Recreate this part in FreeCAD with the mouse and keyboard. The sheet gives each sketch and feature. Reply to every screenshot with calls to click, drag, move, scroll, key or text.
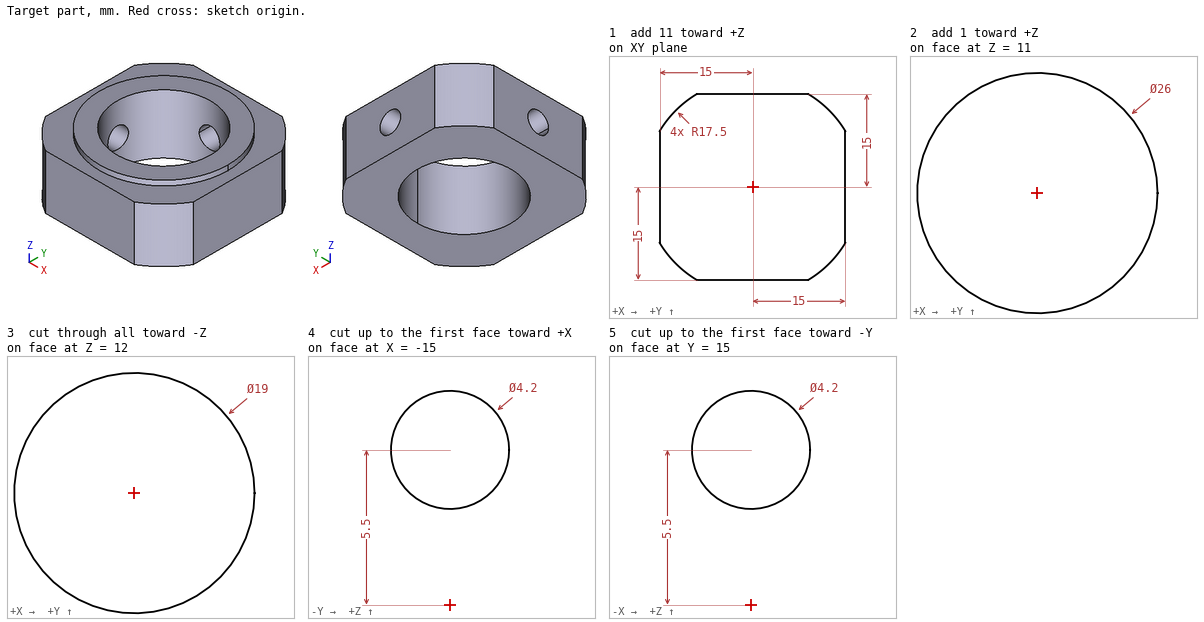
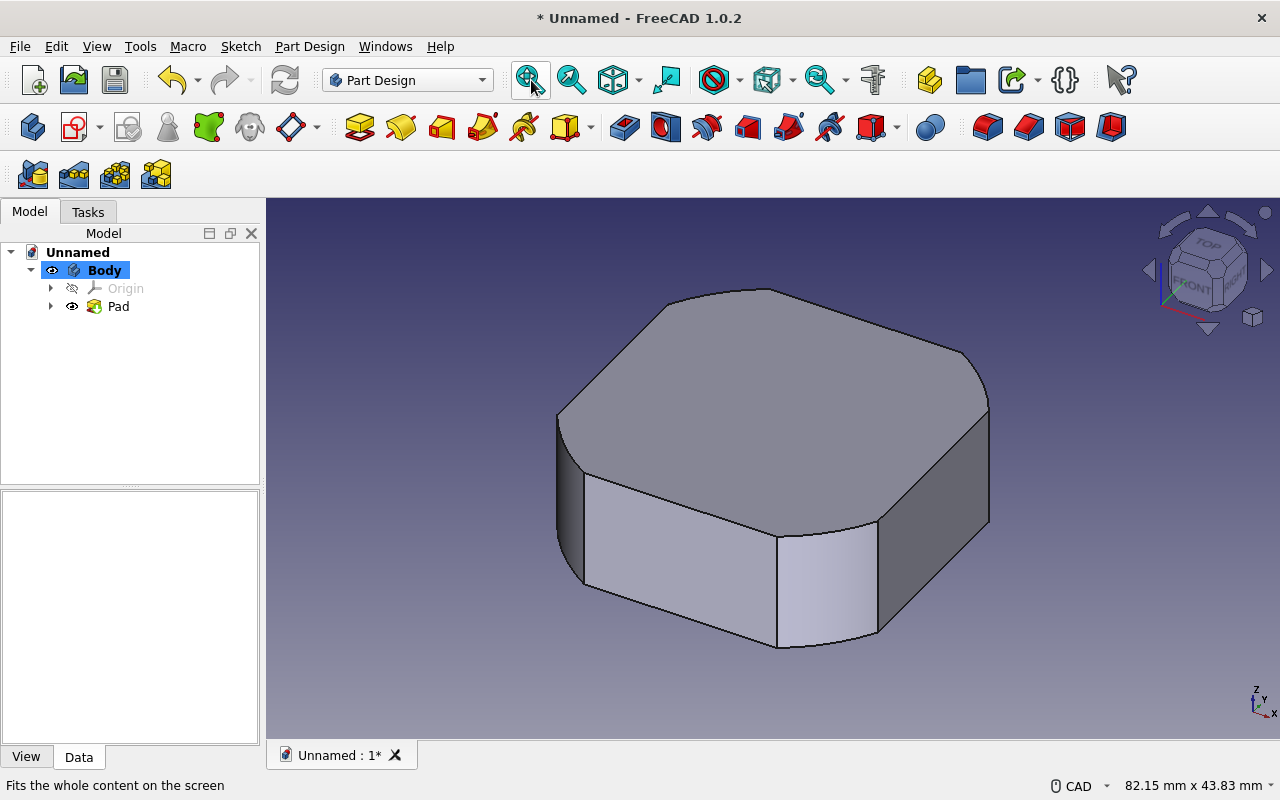
click(773, 412)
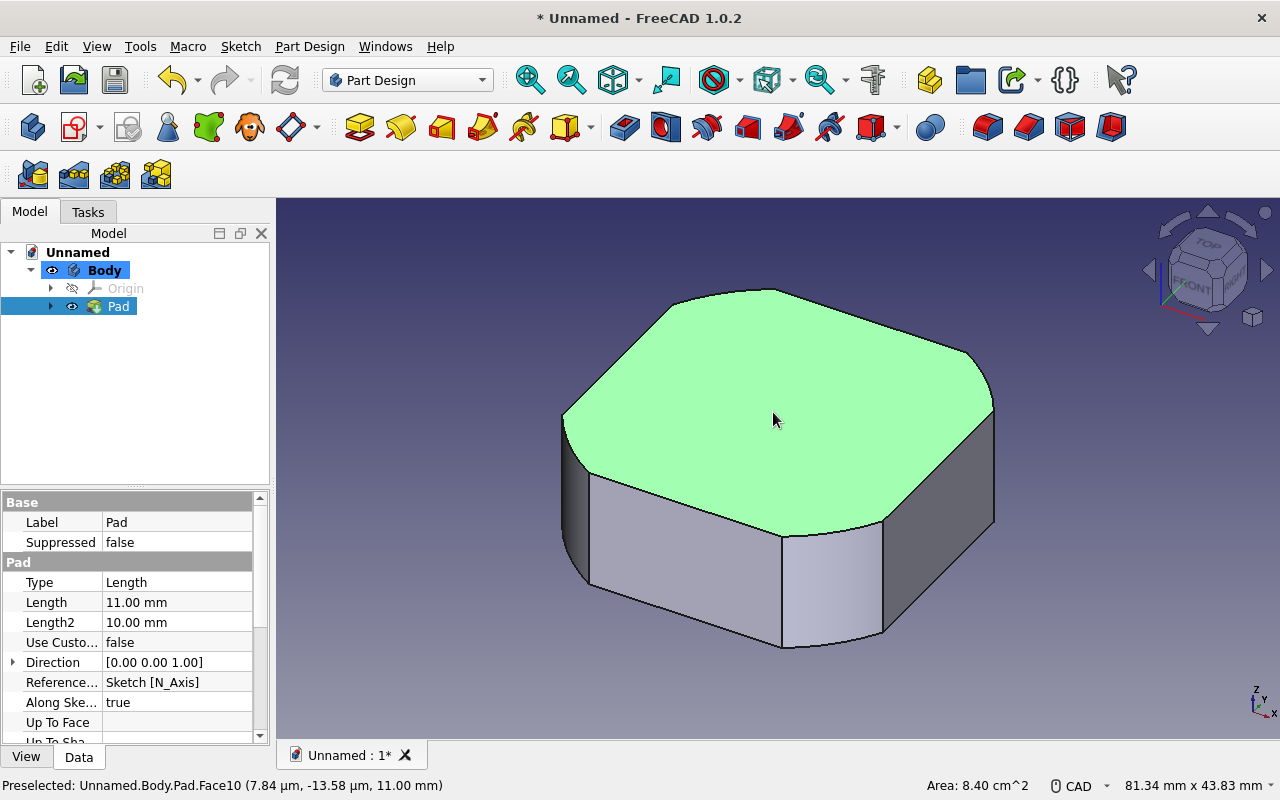
click(74, 128)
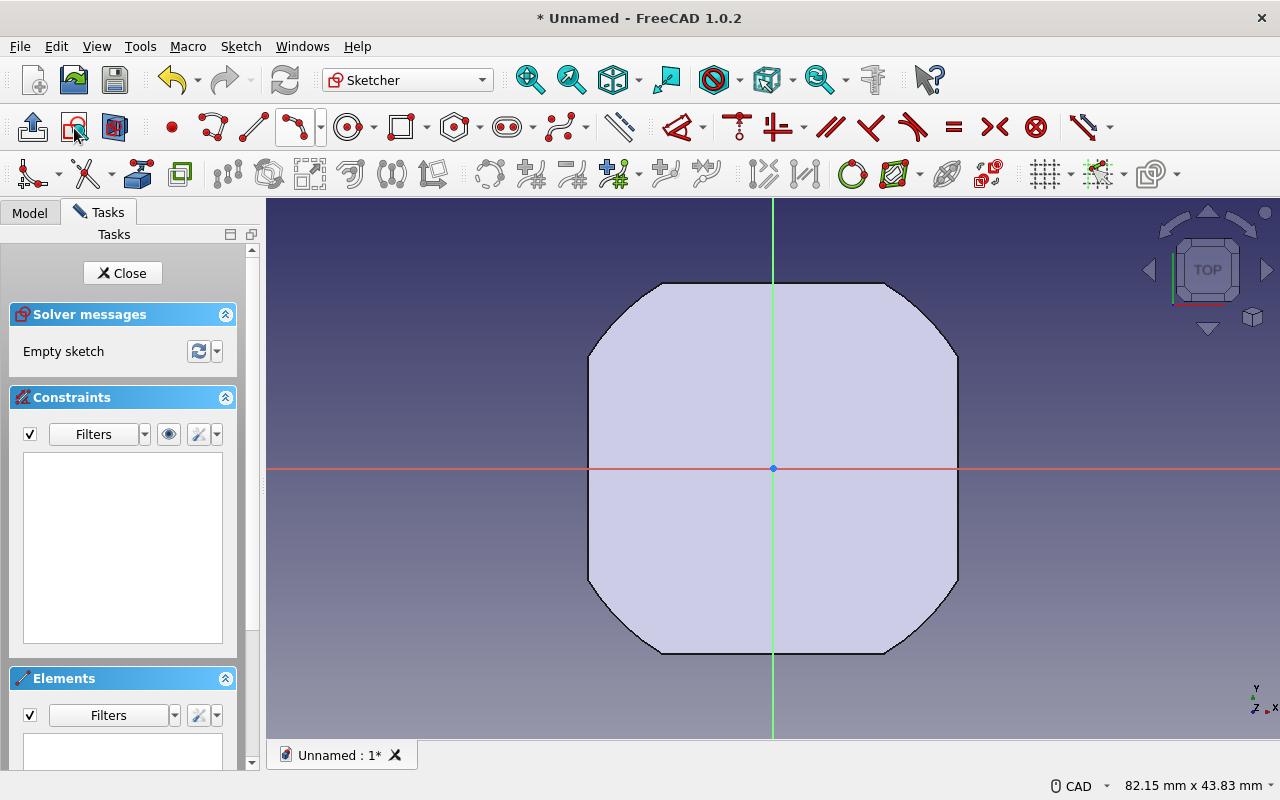
click(348, 128)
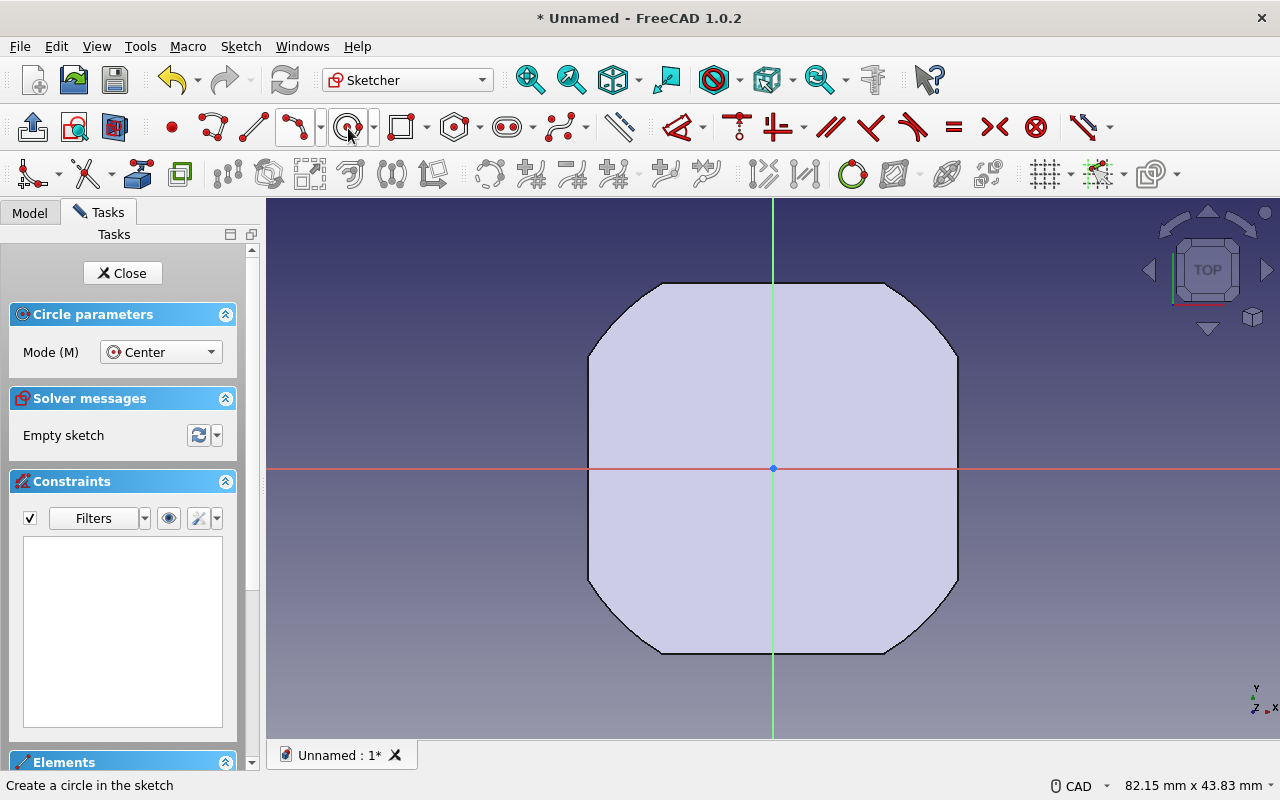
click(773, 468)
click(886, 355)
key(Escape)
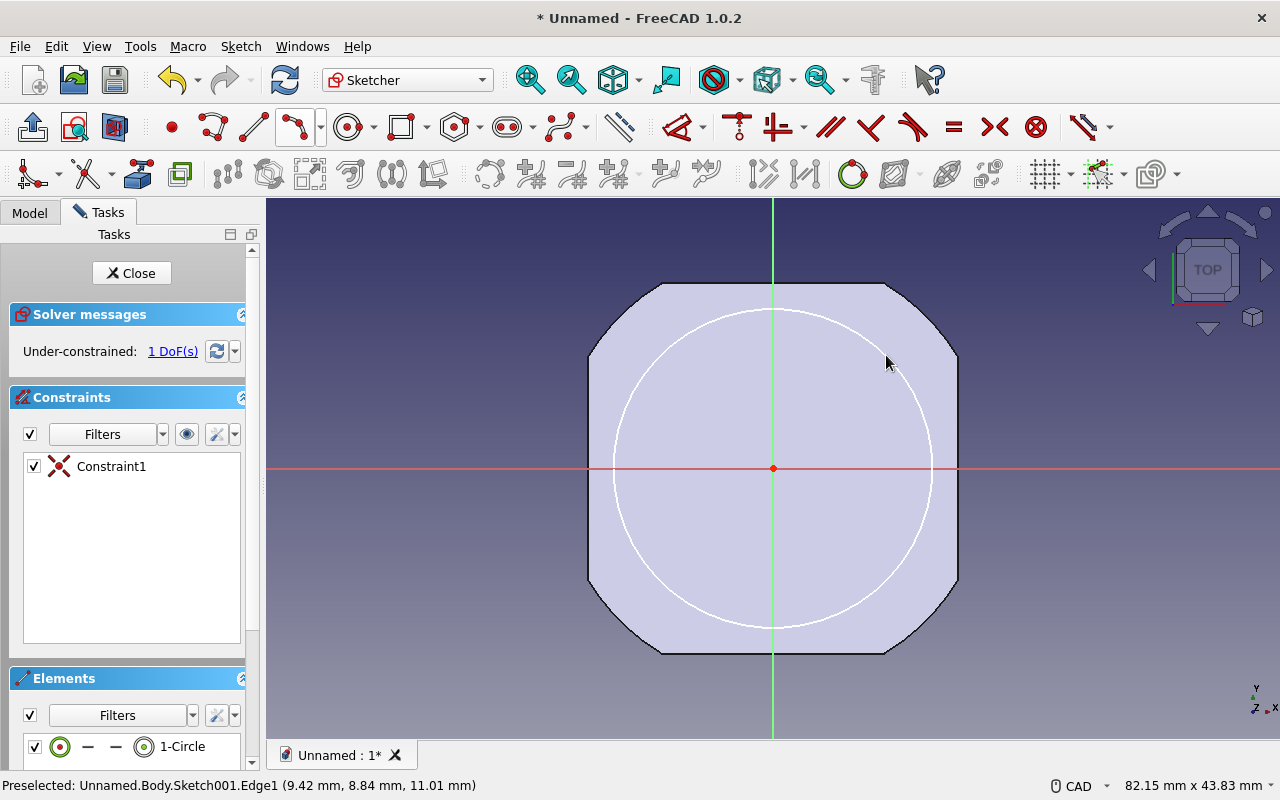
click(676, 128)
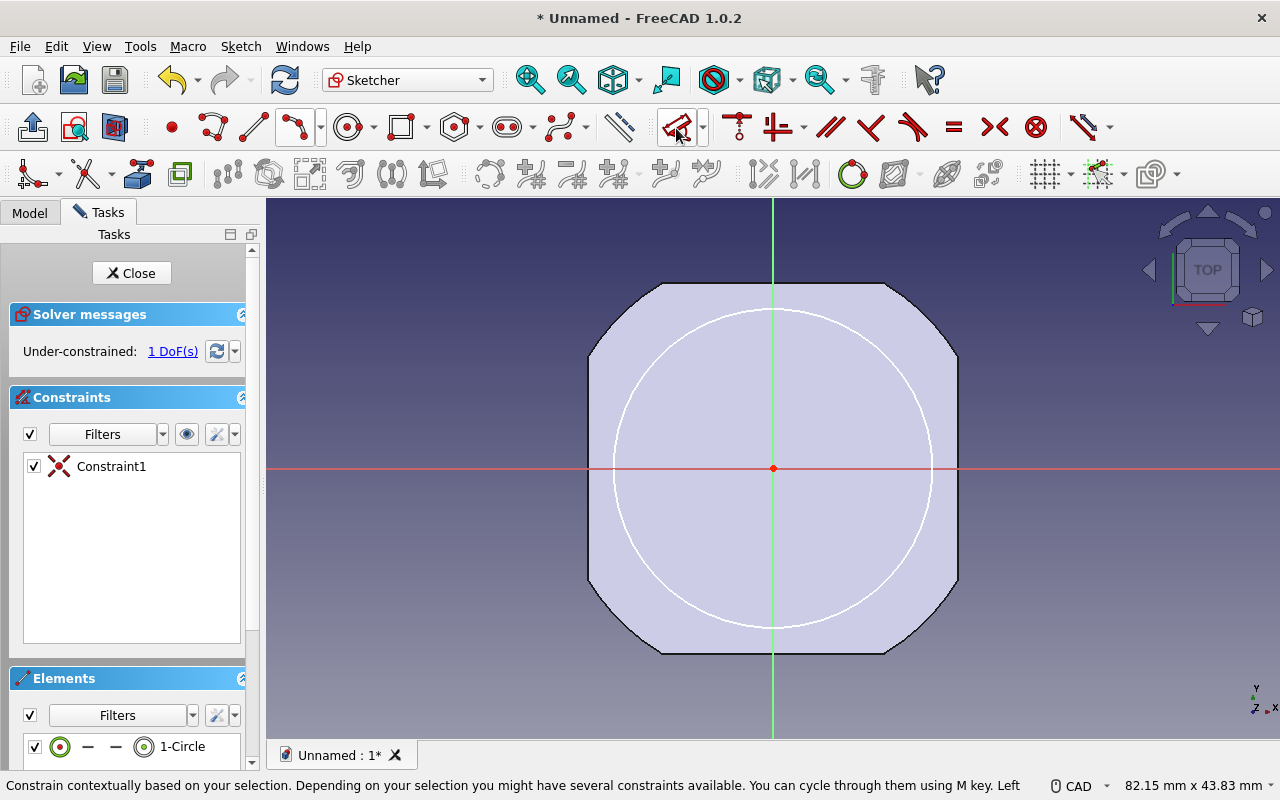
click(885, 355)
click(907, 332)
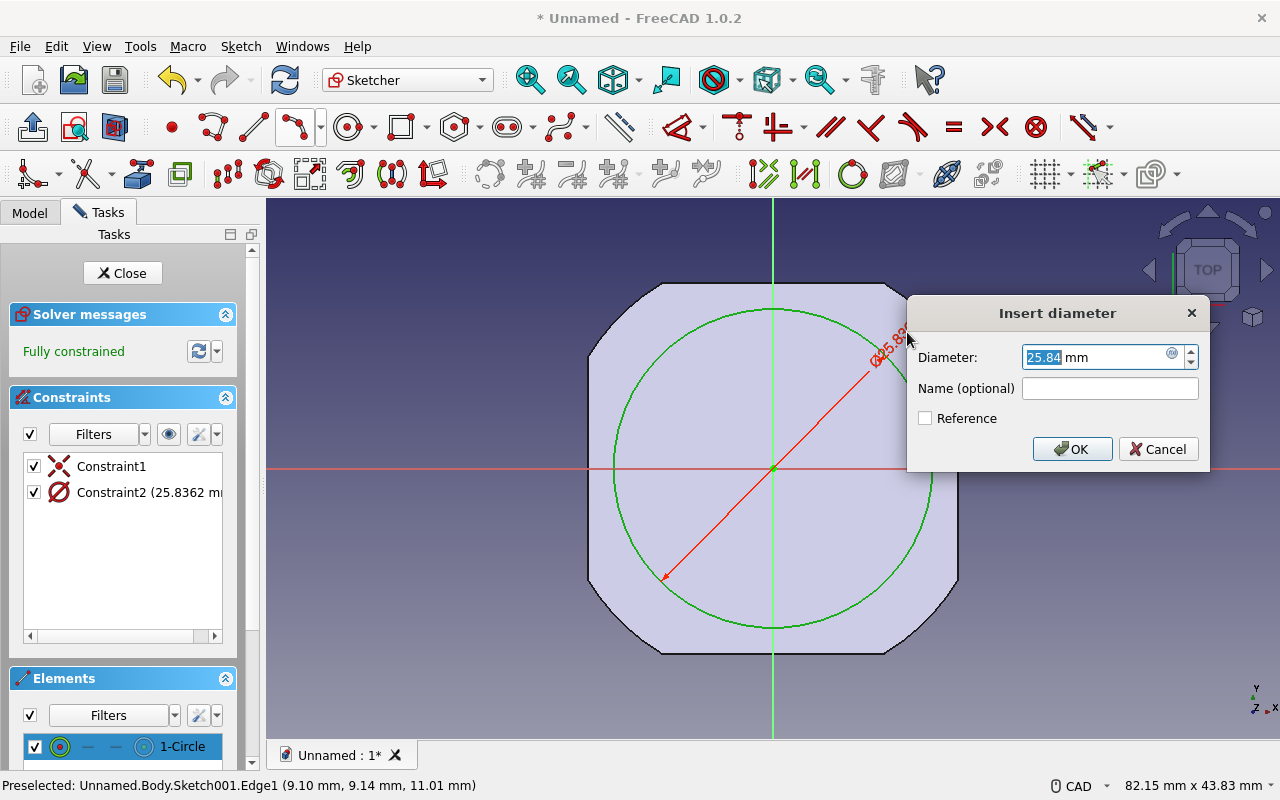
text(26)
key(Return)
key(Escape)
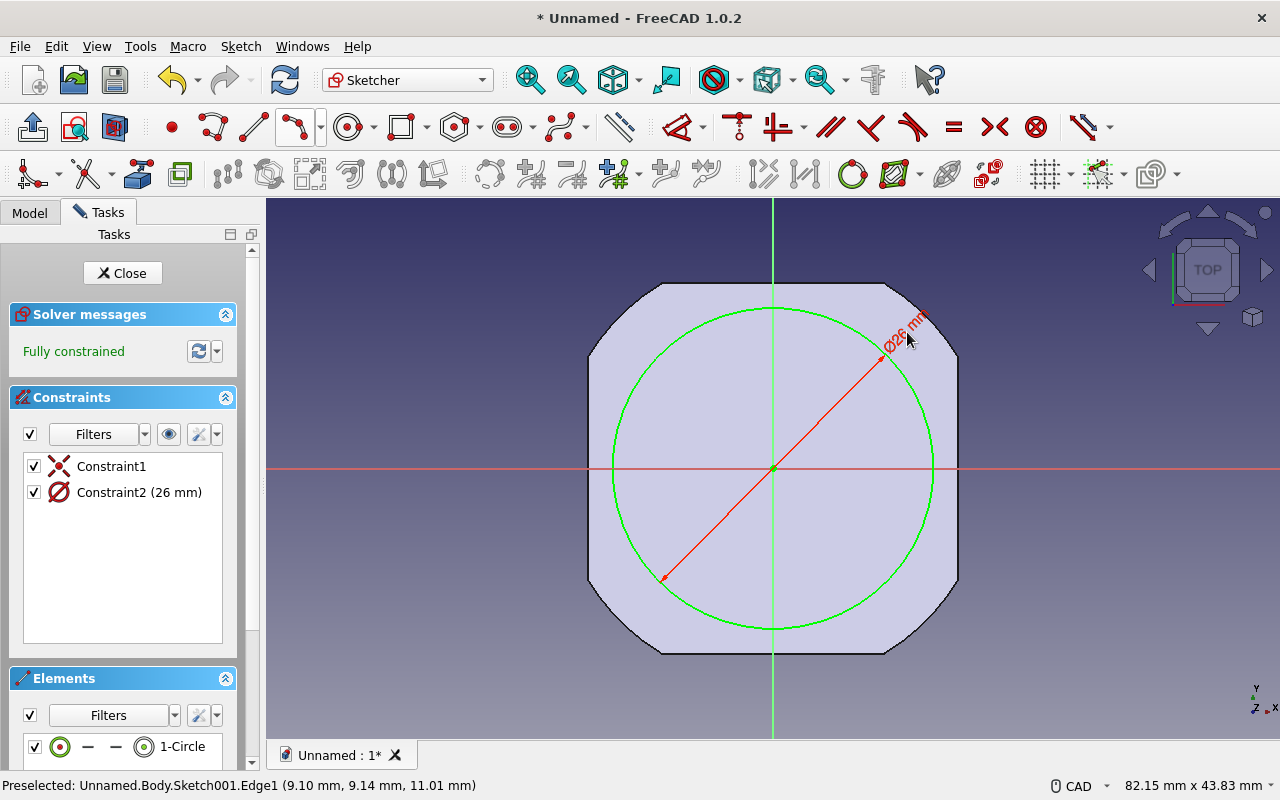
click(123, 273)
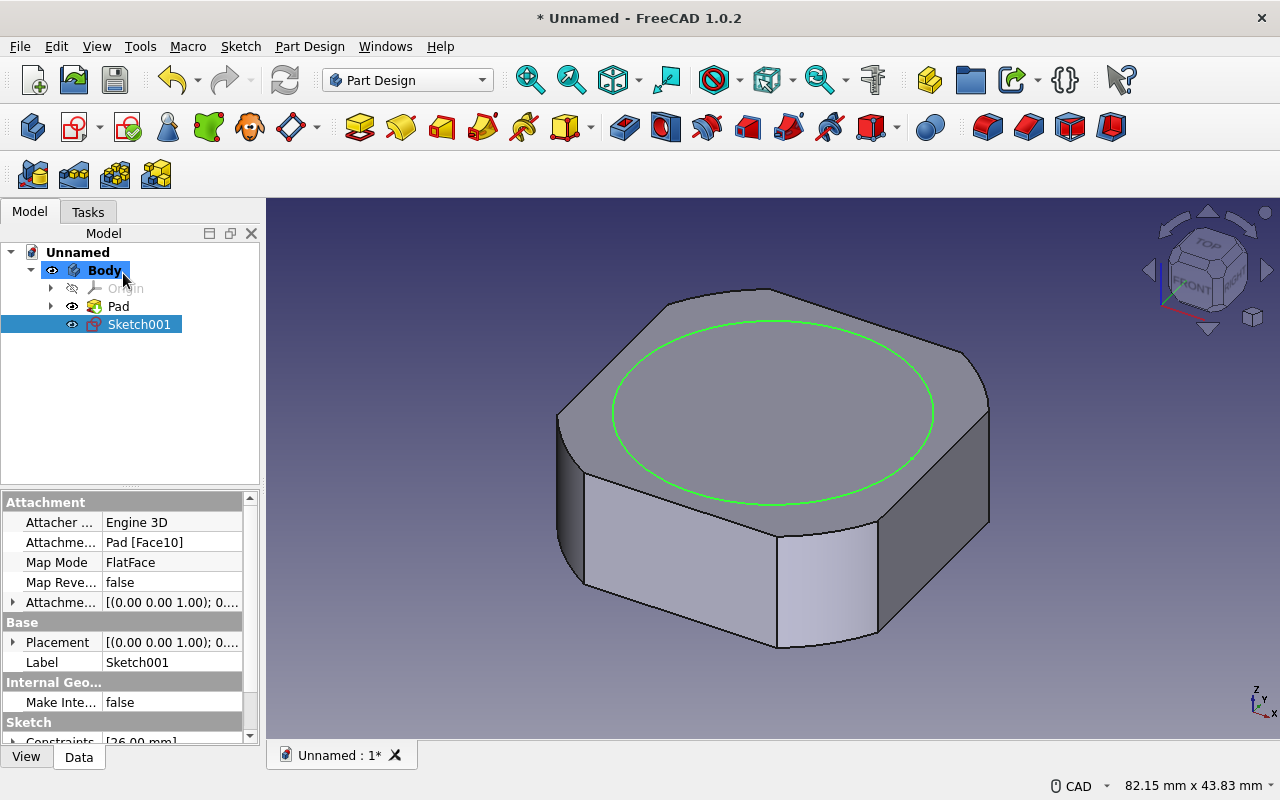
click(360, 128)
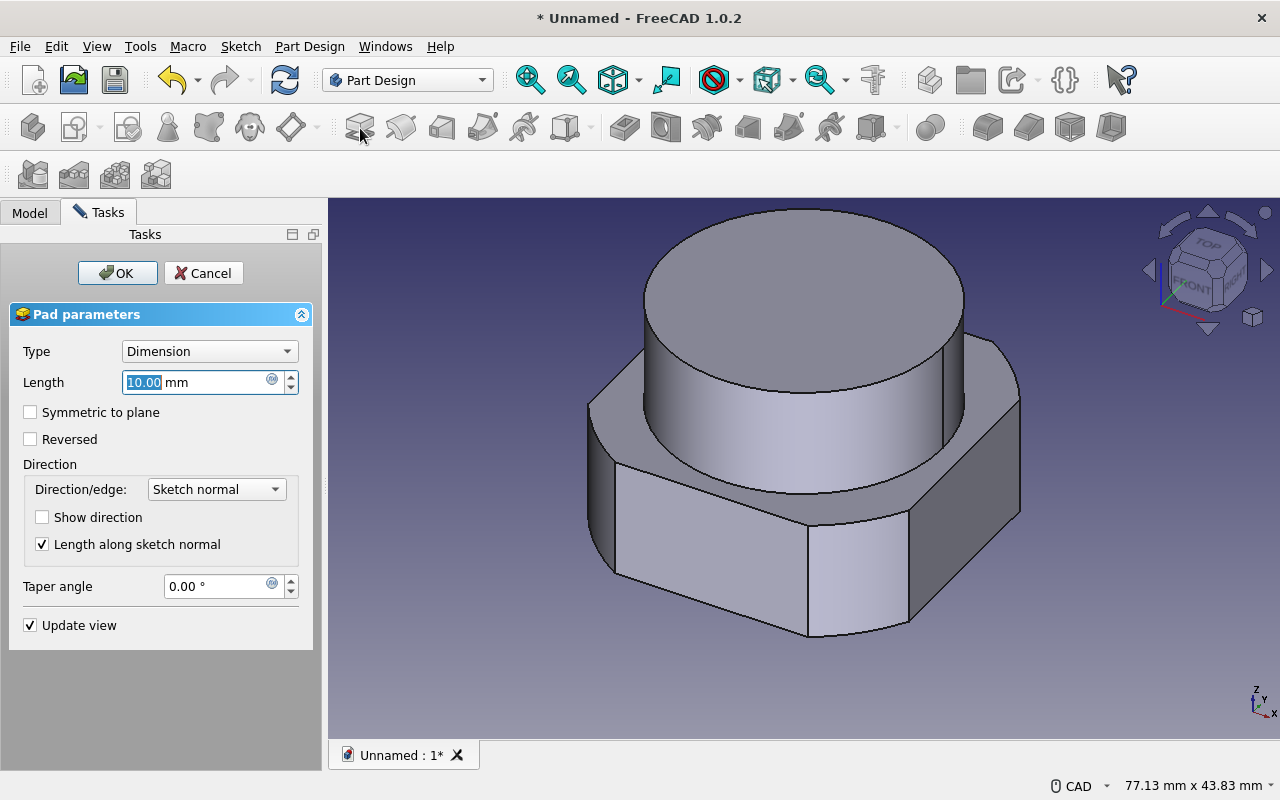
text(1)
key(Tab)